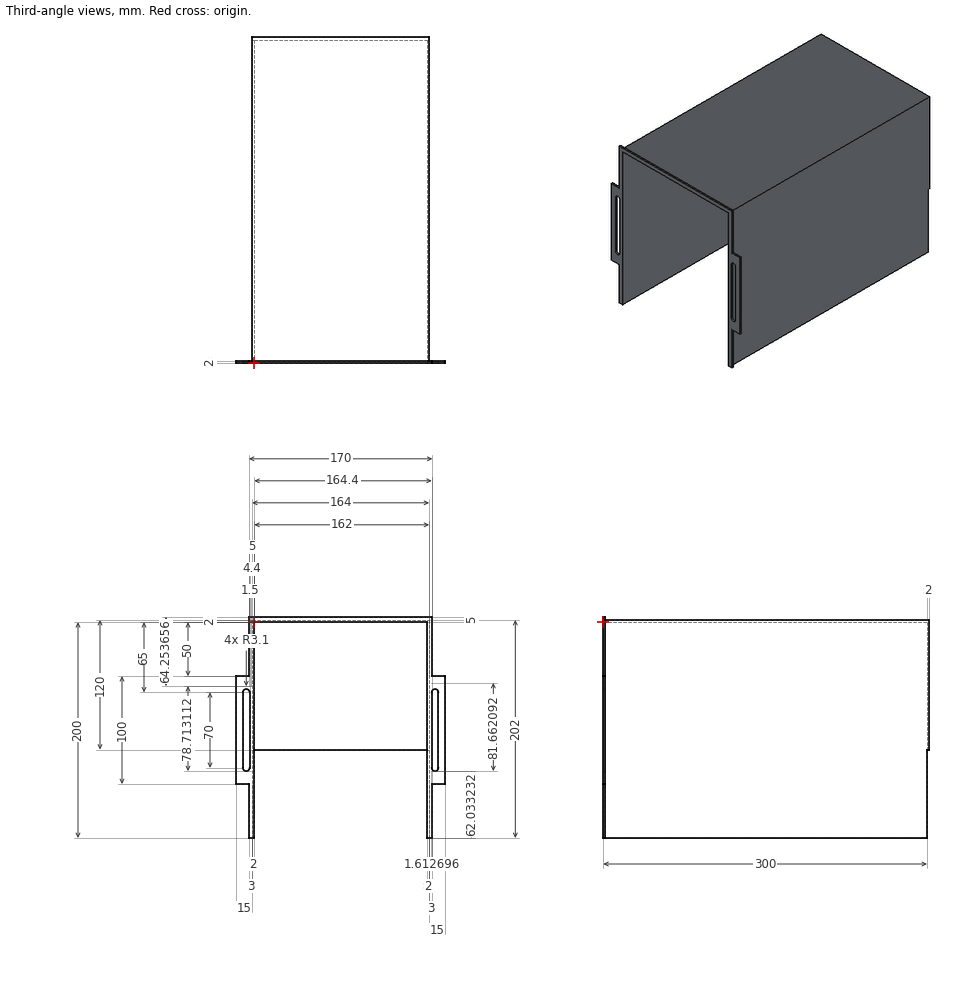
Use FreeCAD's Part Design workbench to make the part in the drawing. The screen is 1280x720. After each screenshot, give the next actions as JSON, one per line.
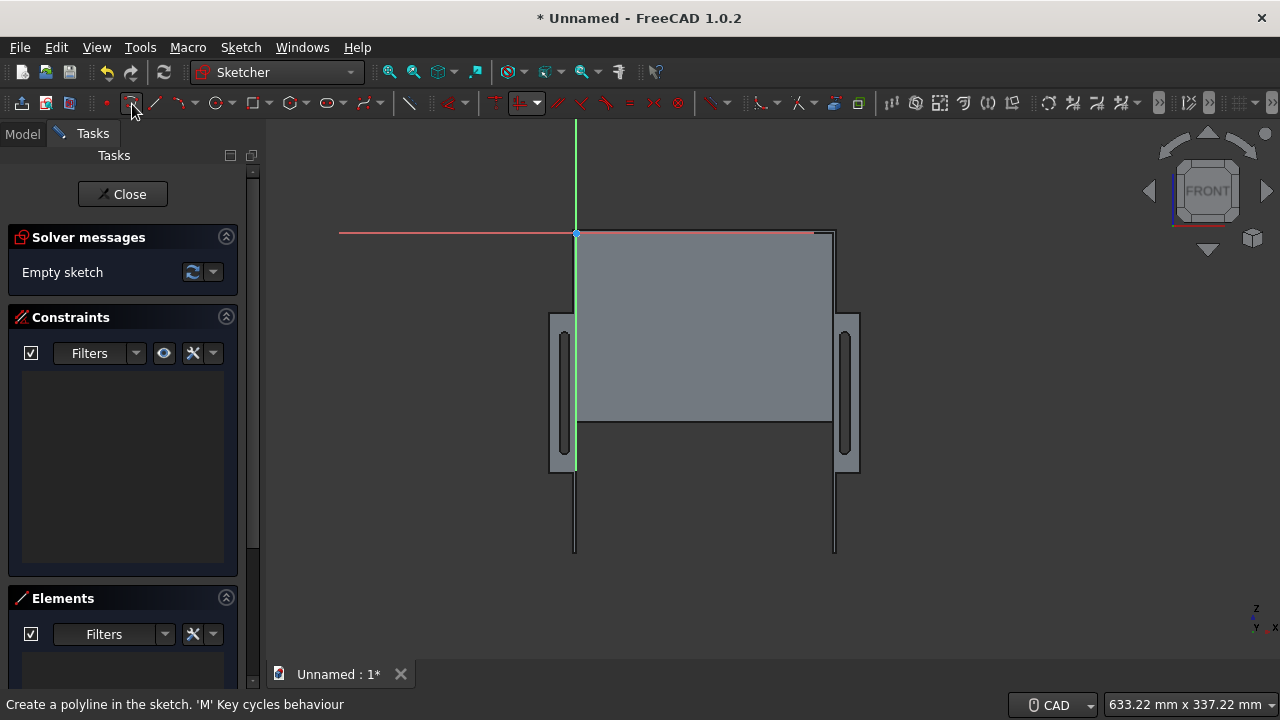
{"action": "scroll", "coordinate": [573, 230], "scroll_direction": "up", "scroll_amount": 9}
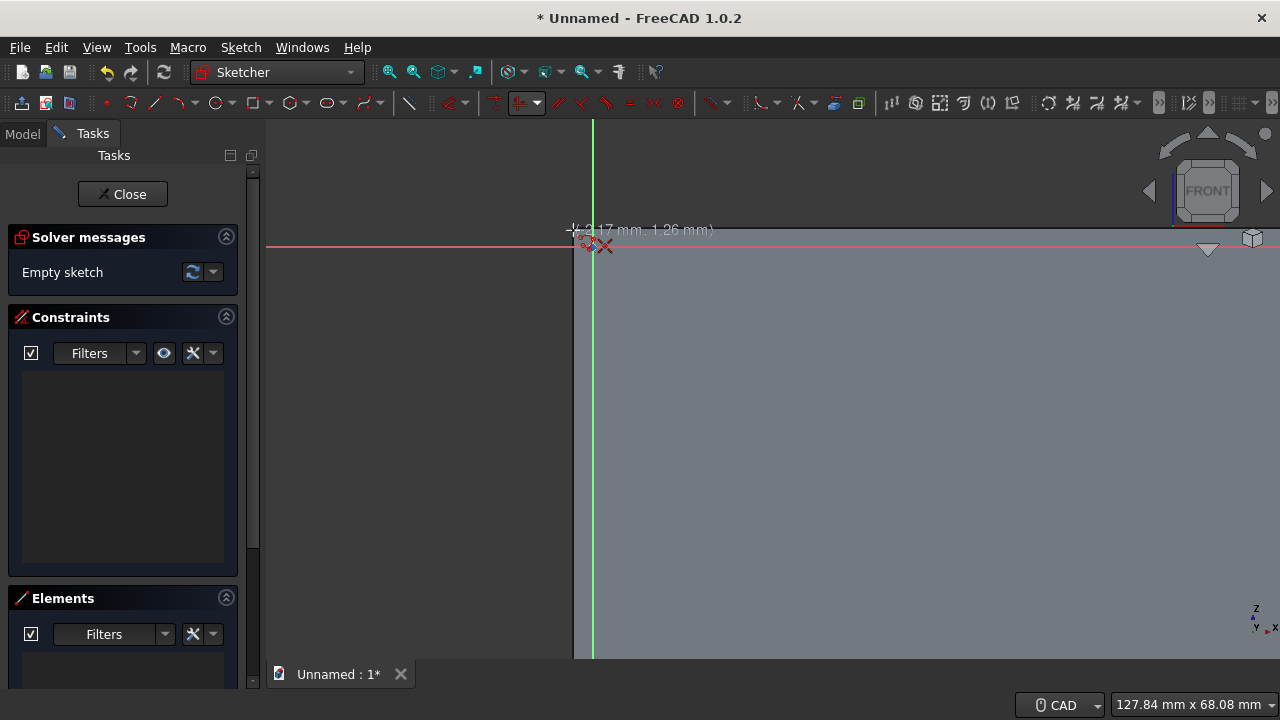
{"action": "left_click", "coordinate": [573, 228]}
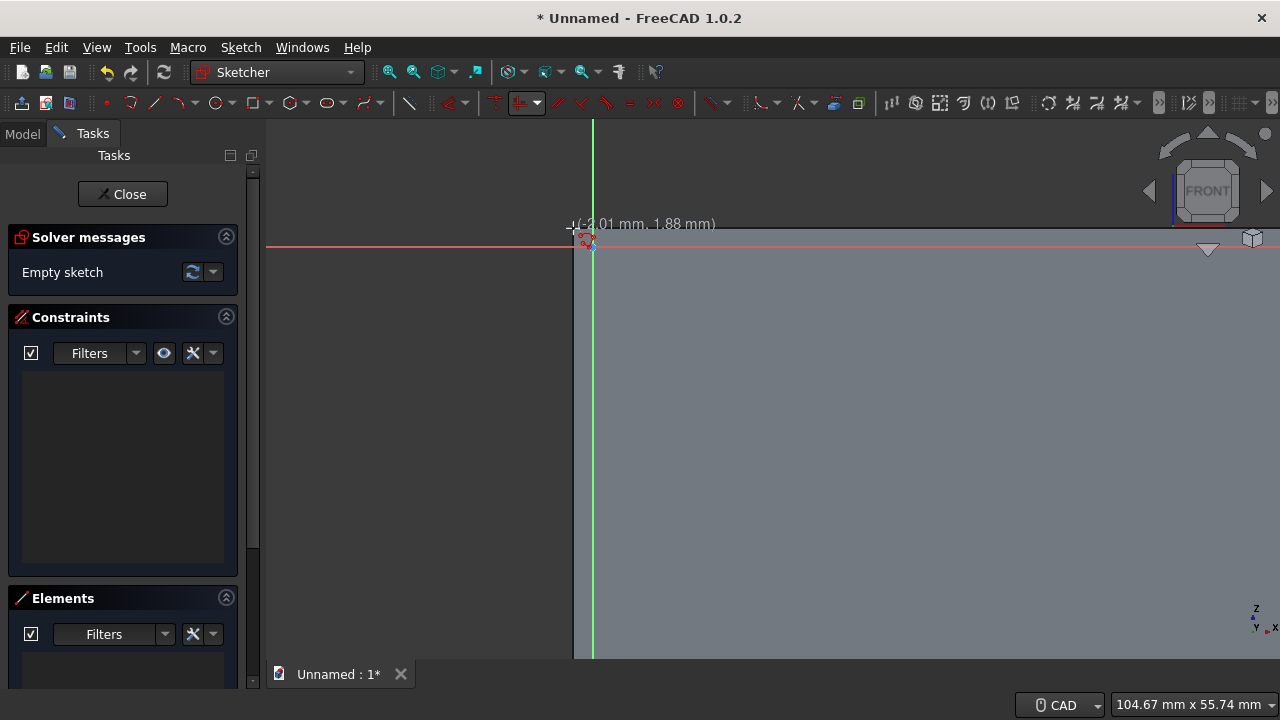
{"action": "scroll", "coordinate": [573, 230], "scroll_direction": "down", "scroll_amount": 9}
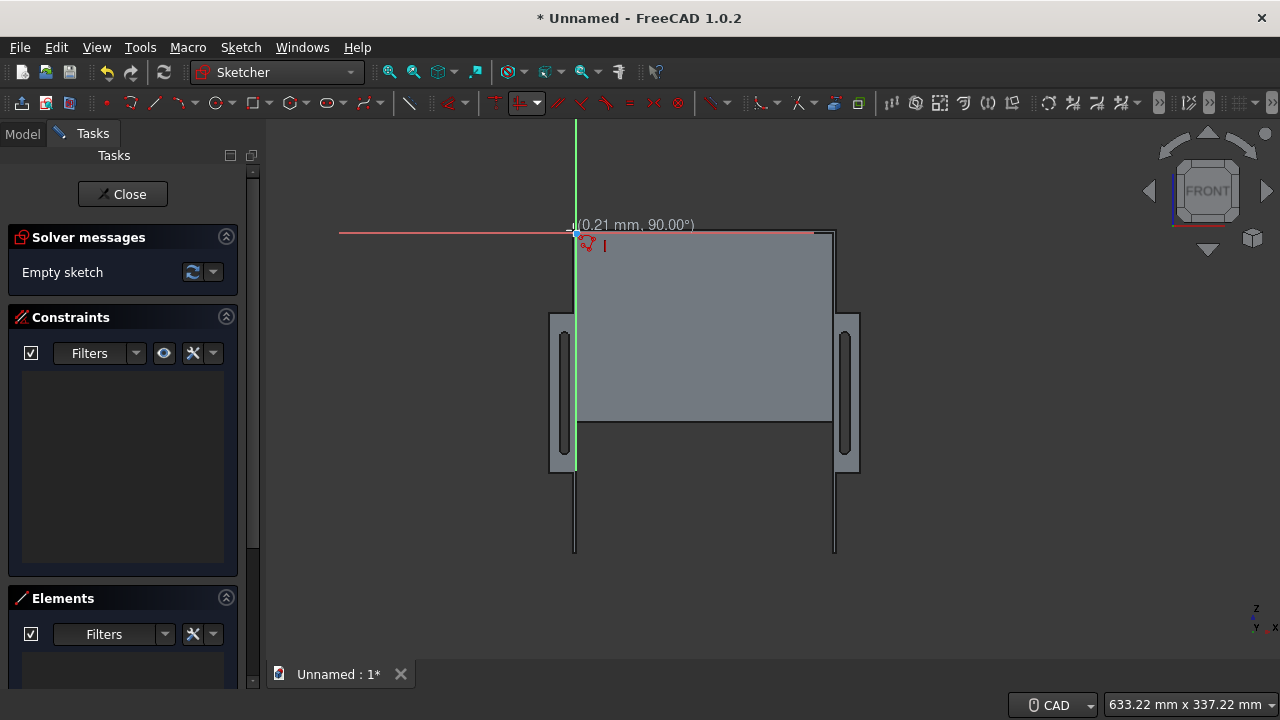
{"action": "scroll", "coordinate": [836, 230], "scroll_direction": "up", "scroll_amount": 9}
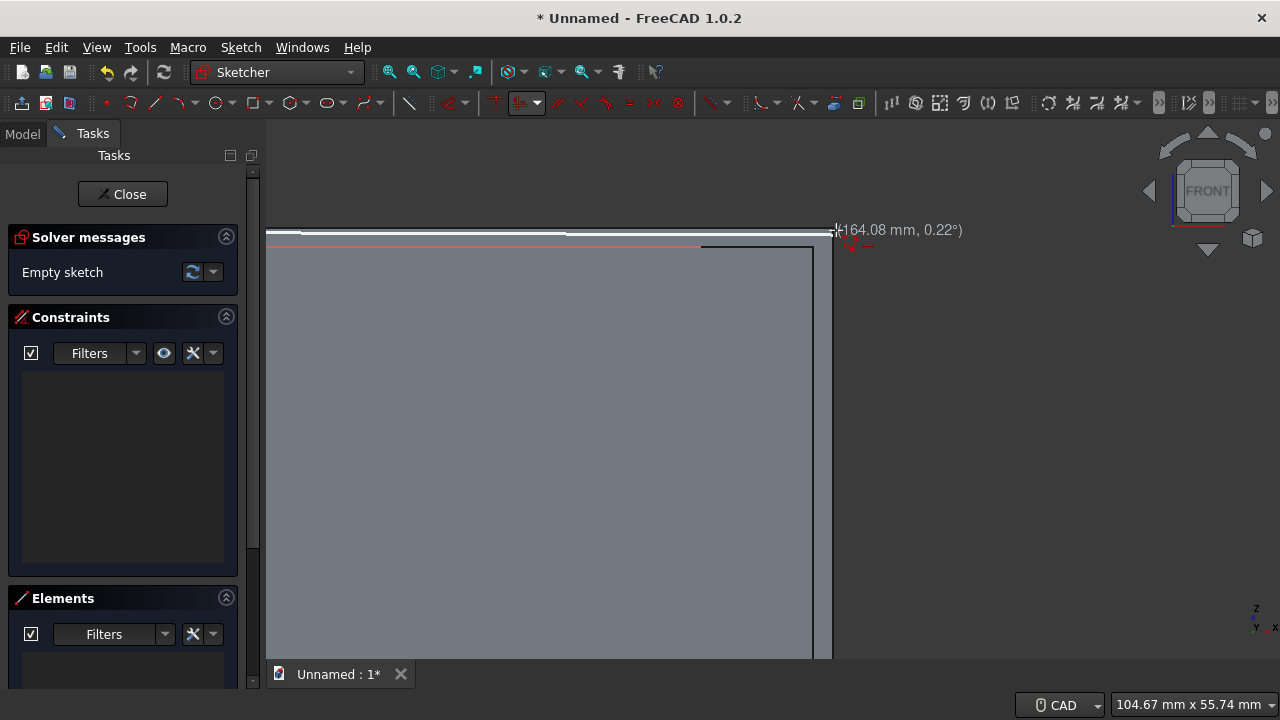
{"action": "left_click", "coordinate": [833, 228]}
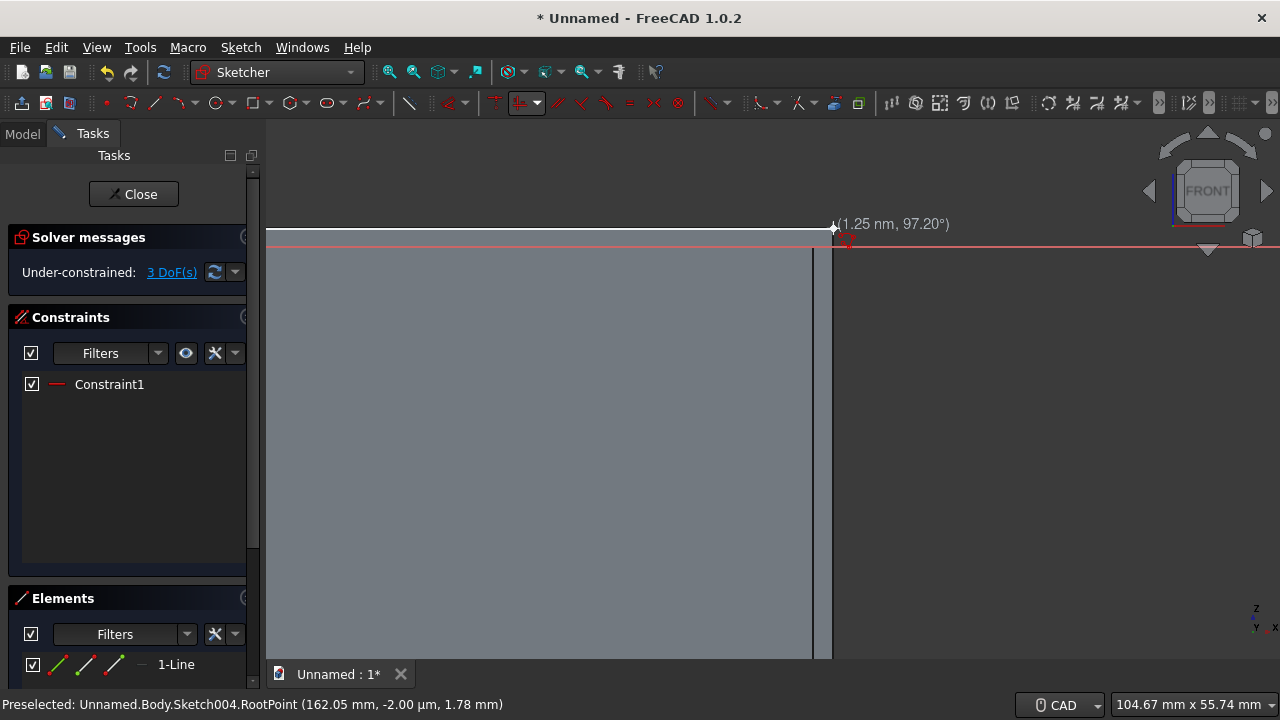
{"action": "scroll", "coordinate": [836, 230], "scroll_direction": "down", "scroll_amount": 9}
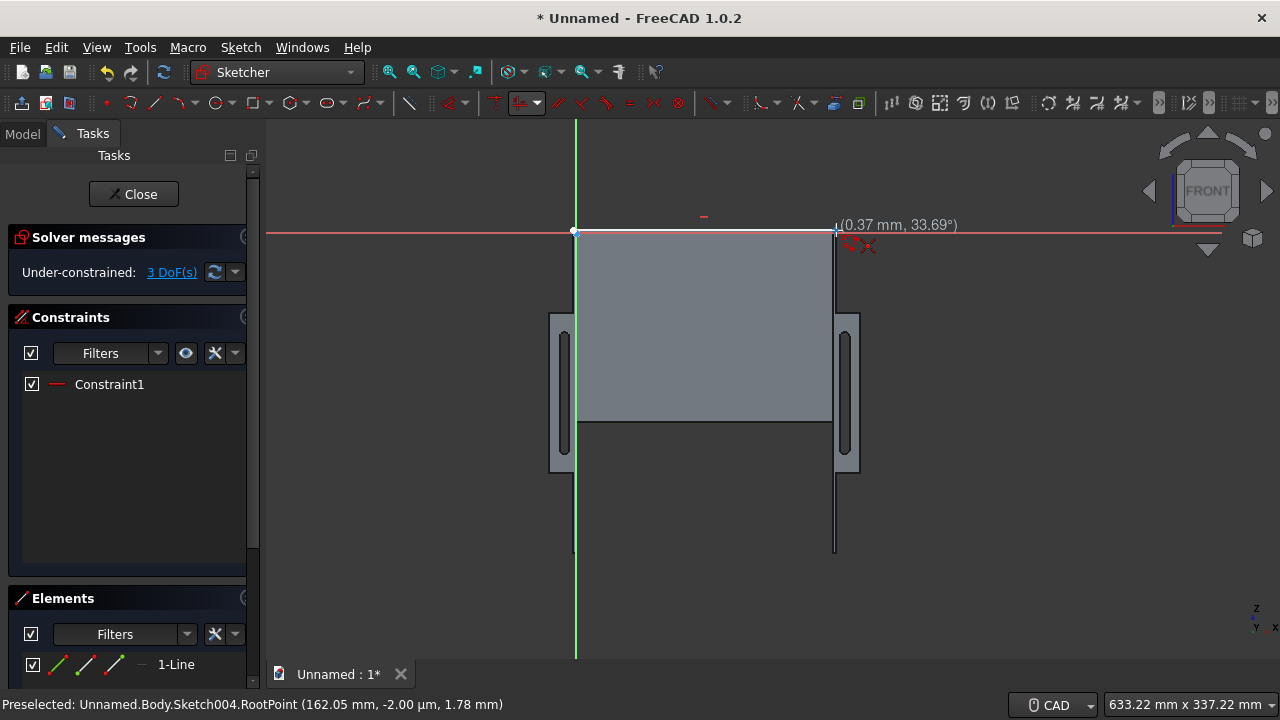
{"action": "left_click", "coordinate": [836, 553]}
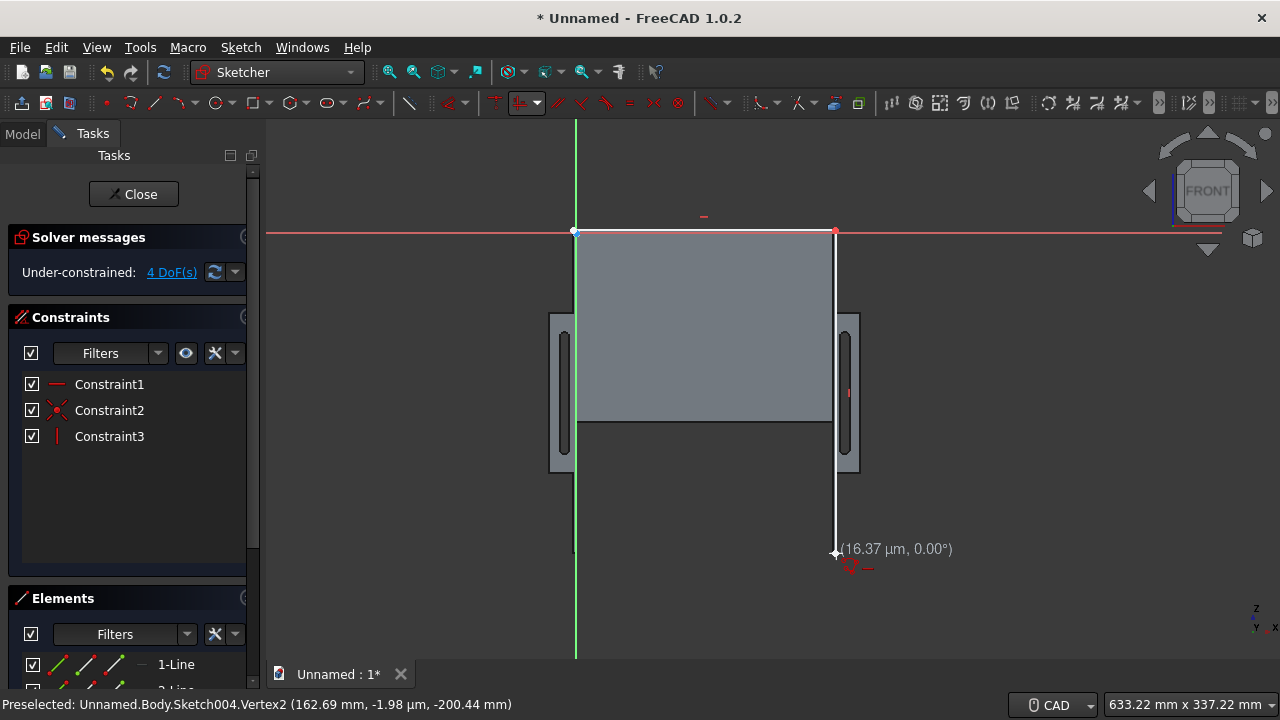
{"action": "scroll", "coordinate": [841, 553], "scroll_direction": "up", "scroll_amount": 6}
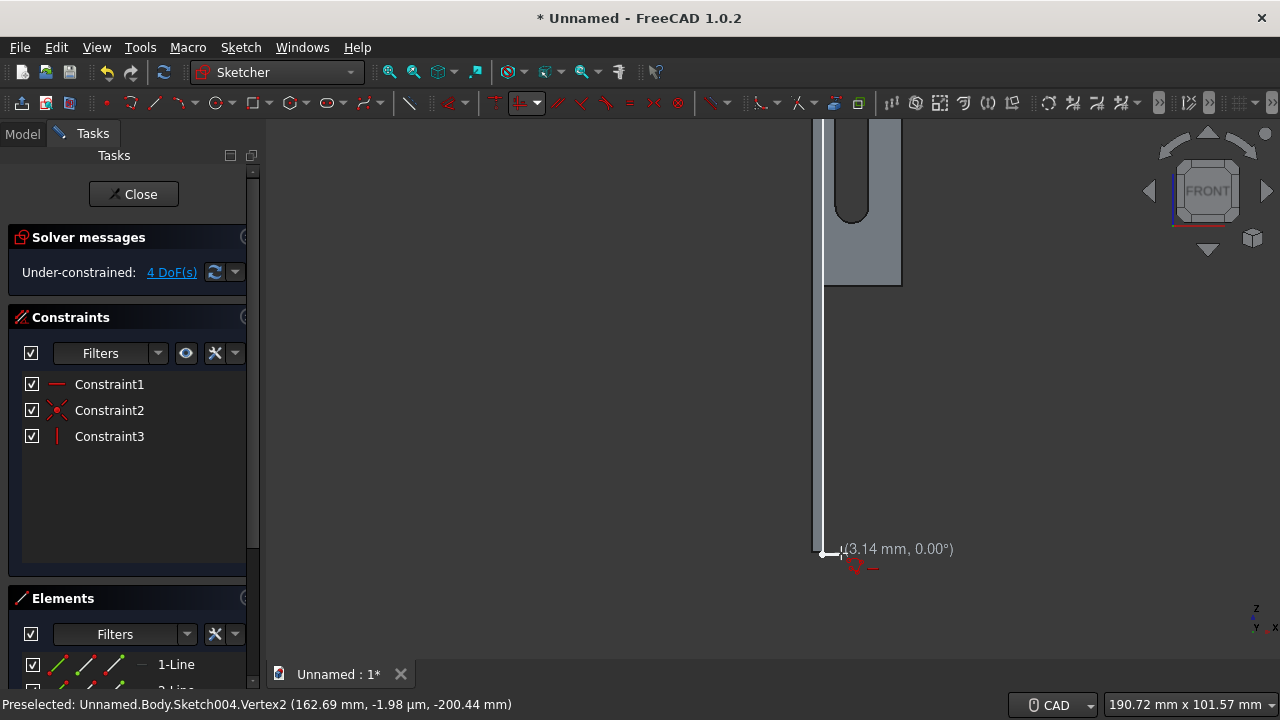
{"action": "left_click", "coordinate": [839, 551]}
{"action": "left_click", "coordinate": [839, 222]}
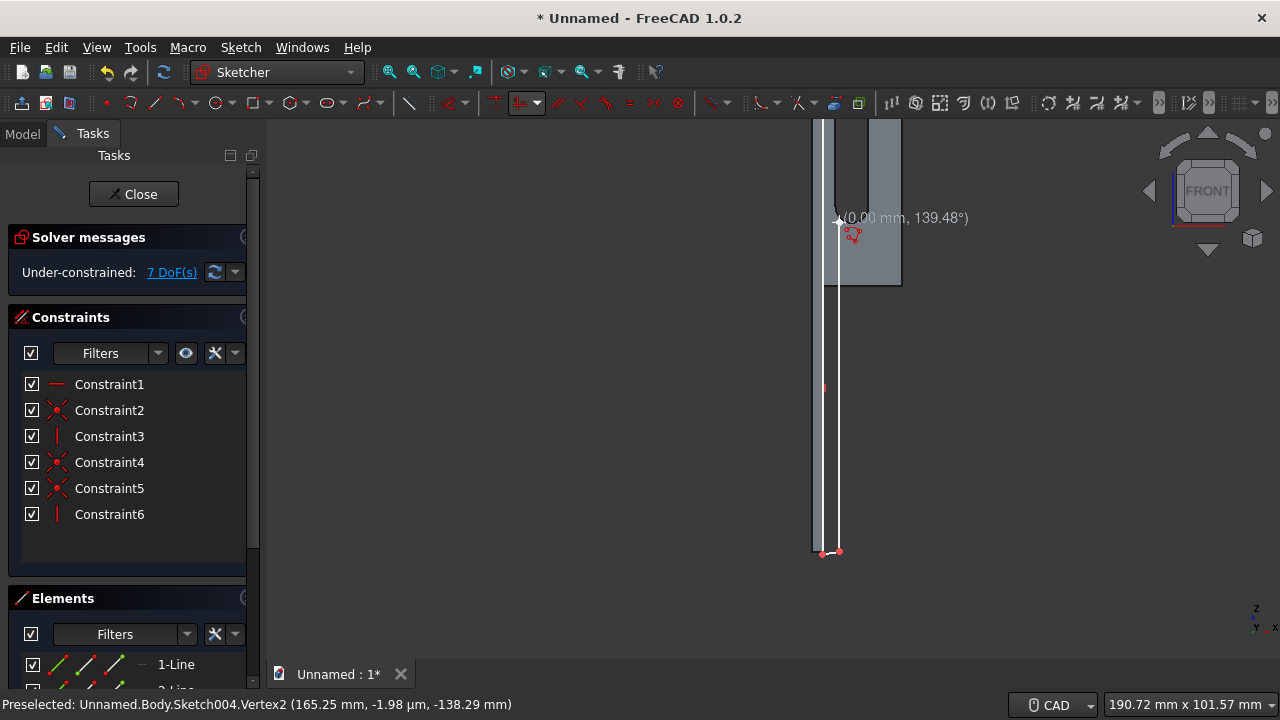
{"action": "scroll", "coordinate": [830, 222], "scroll_direction": "up", "scroll_amount": 4}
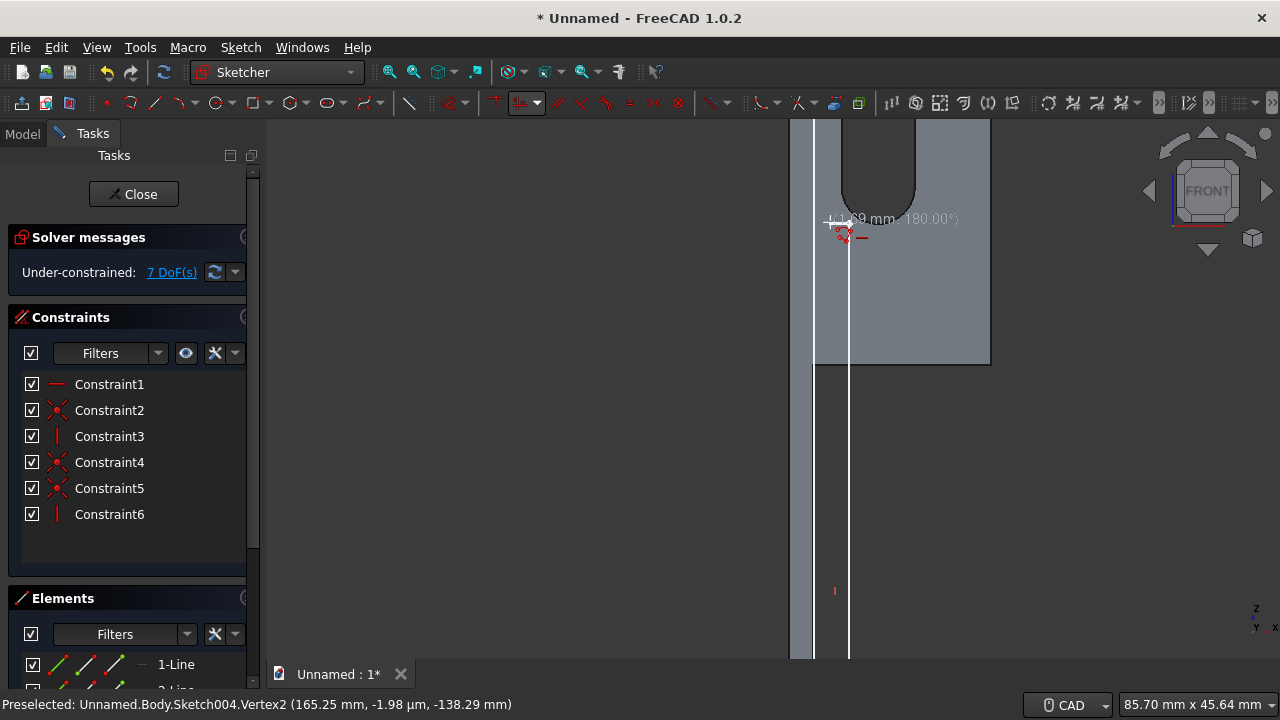
{"action": "left_click", "coordinate": [830, 222]}